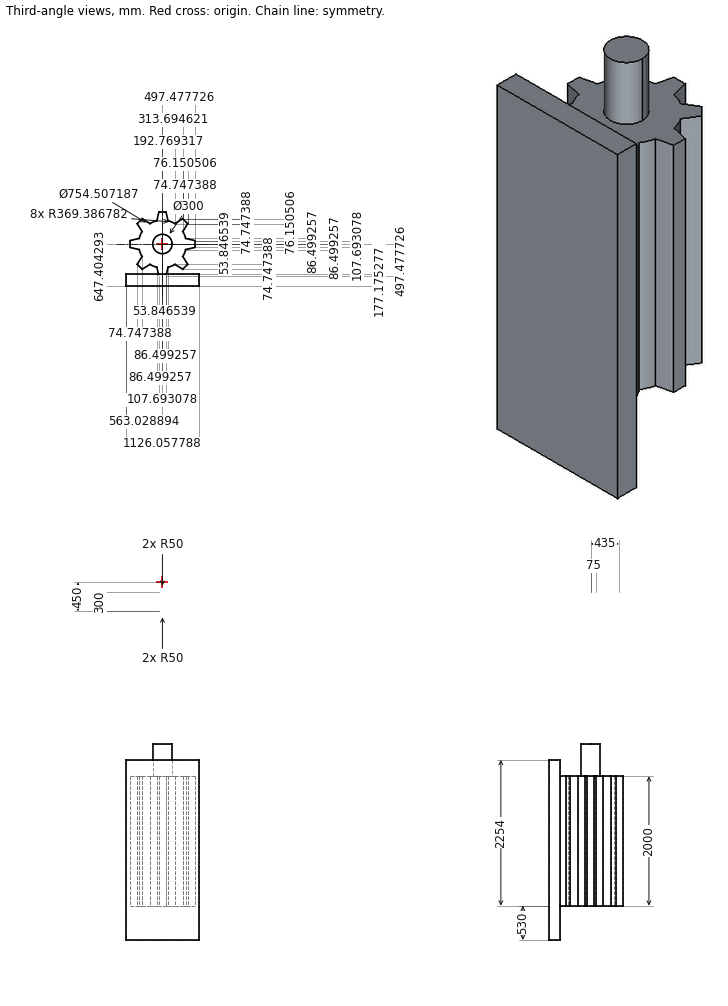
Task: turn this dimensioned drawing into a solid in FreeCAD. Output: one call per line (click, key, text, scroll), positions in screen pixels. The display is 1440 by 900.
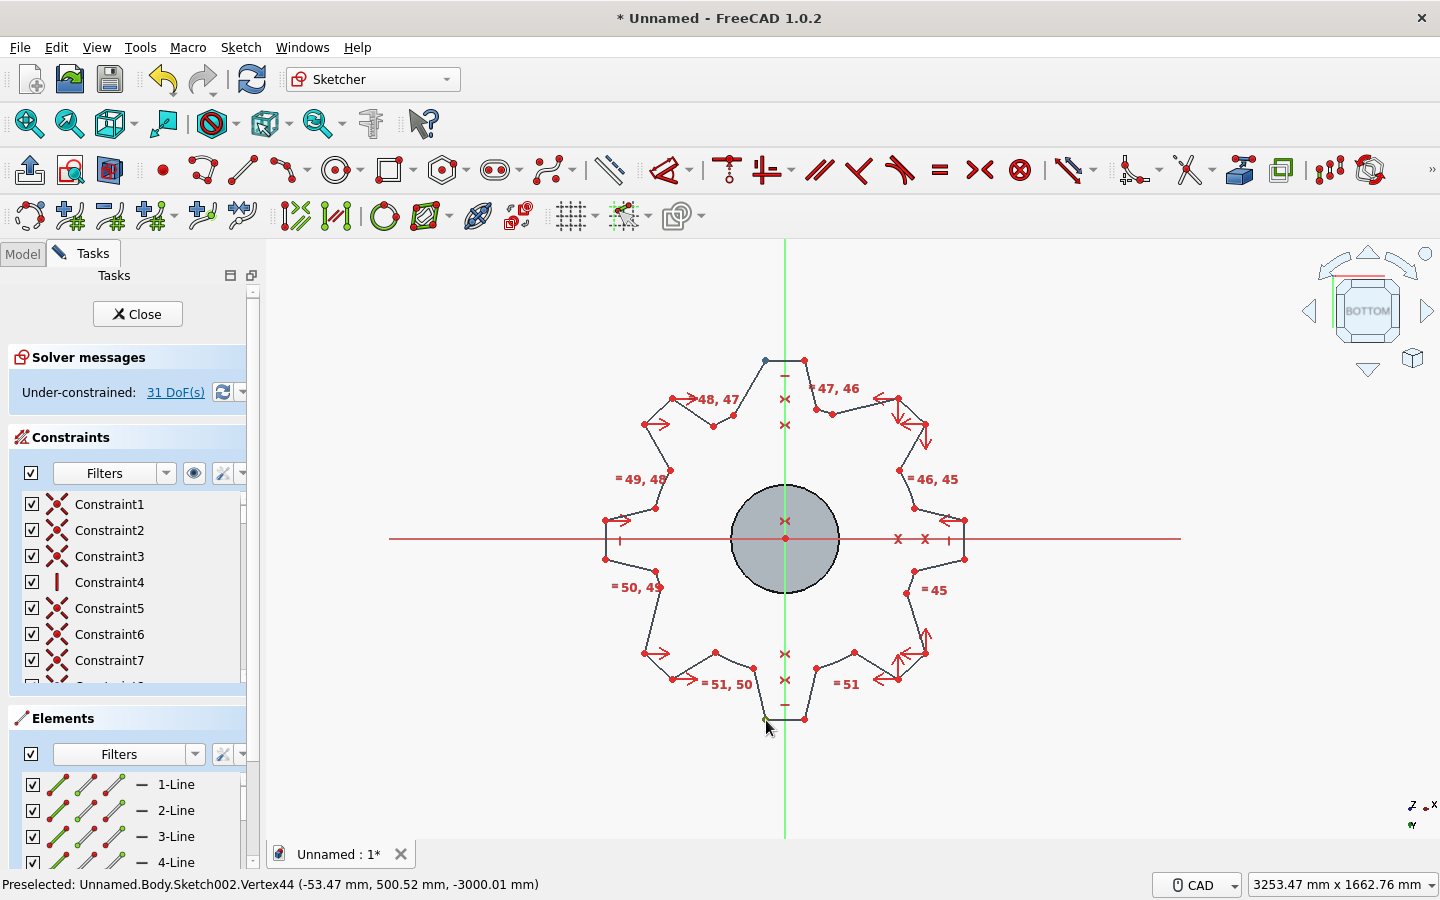
click(434, 539)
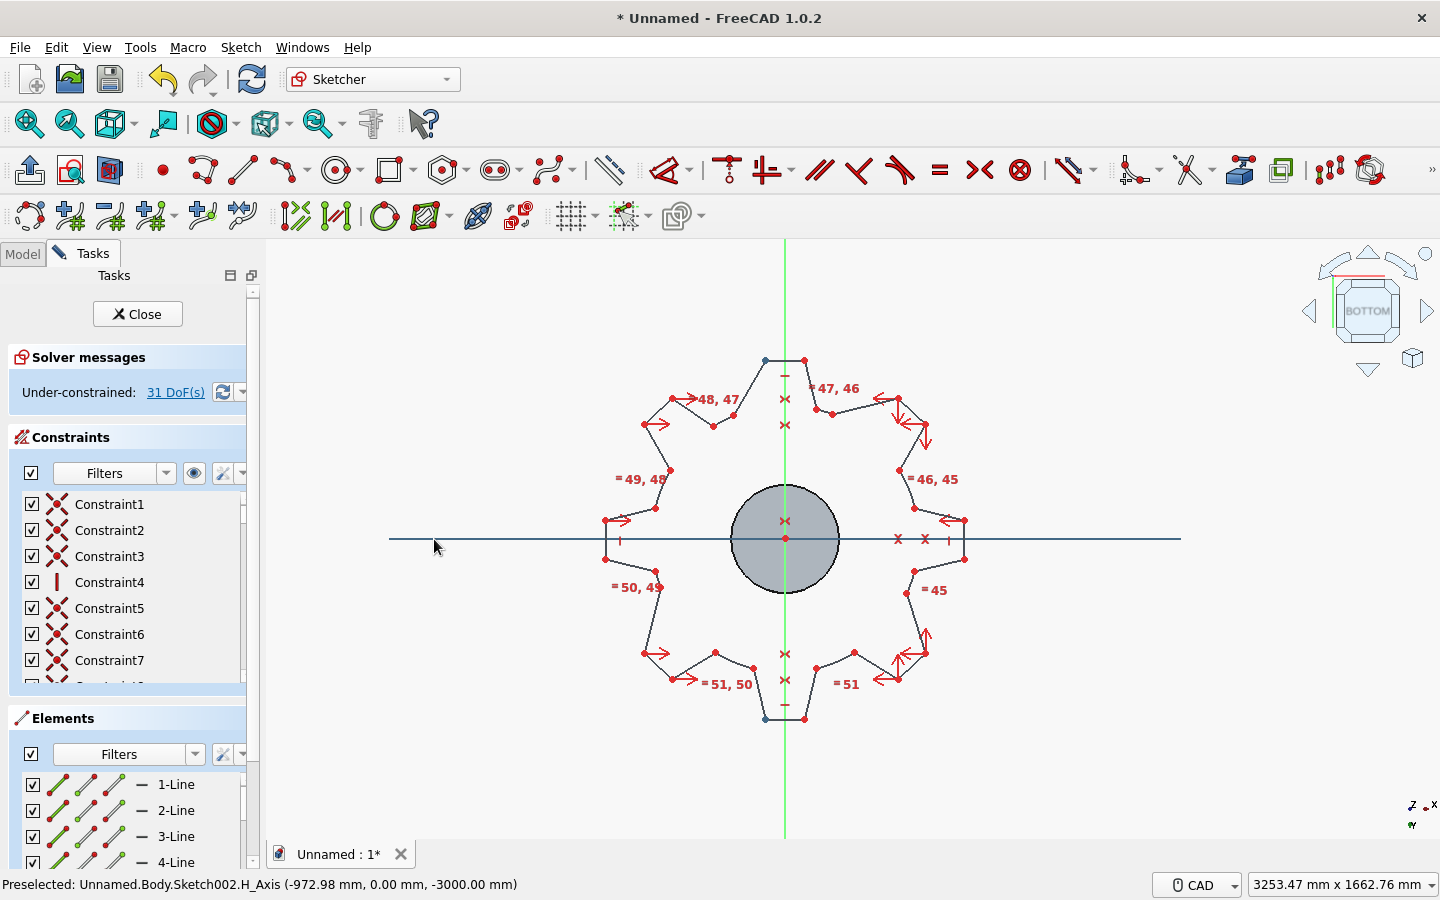
click(980, 170)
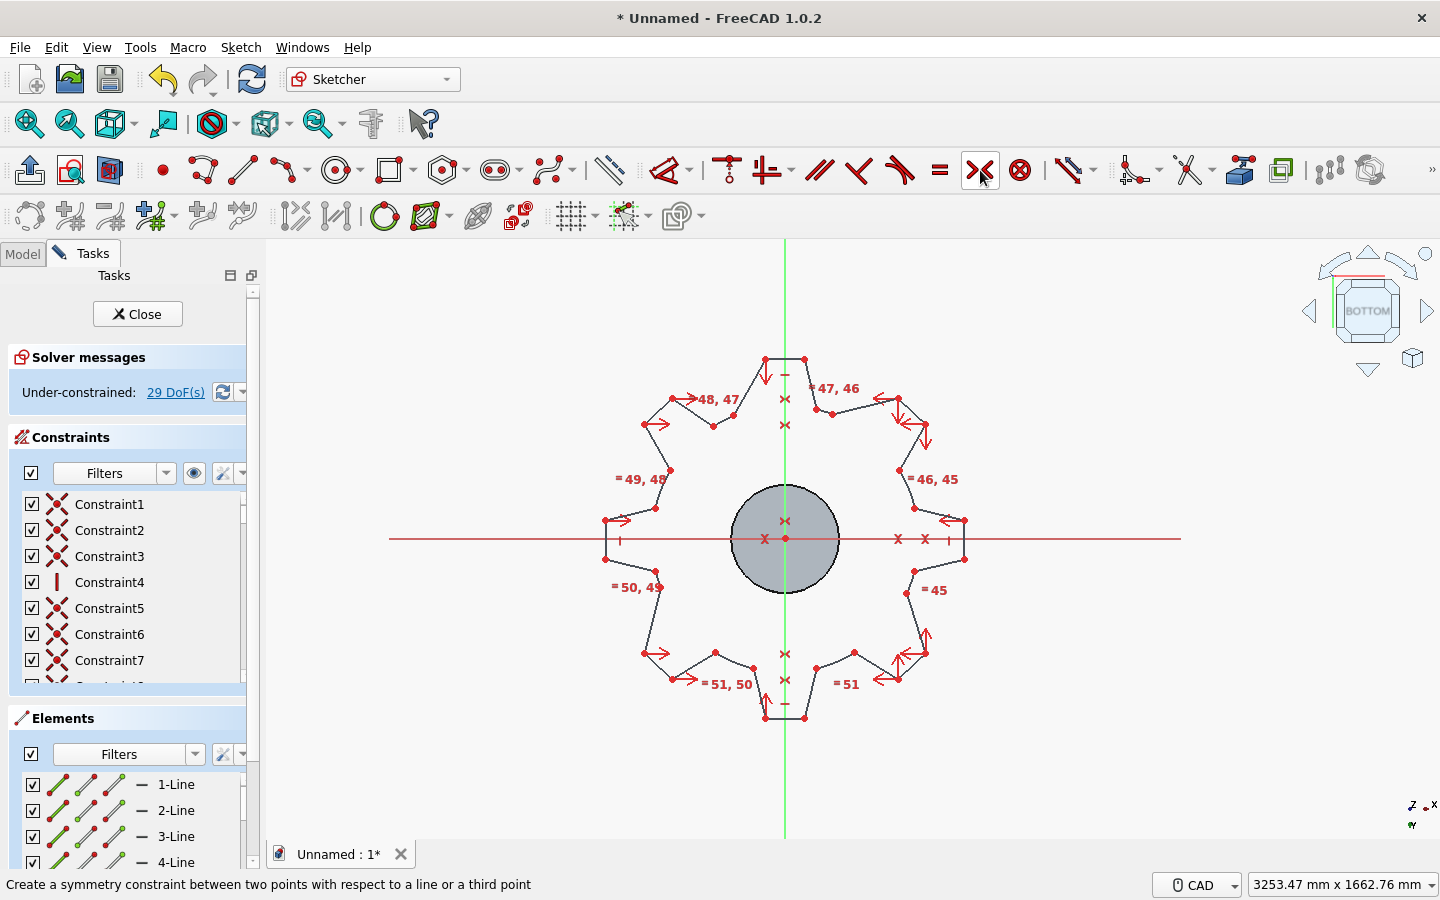
click(664, 170)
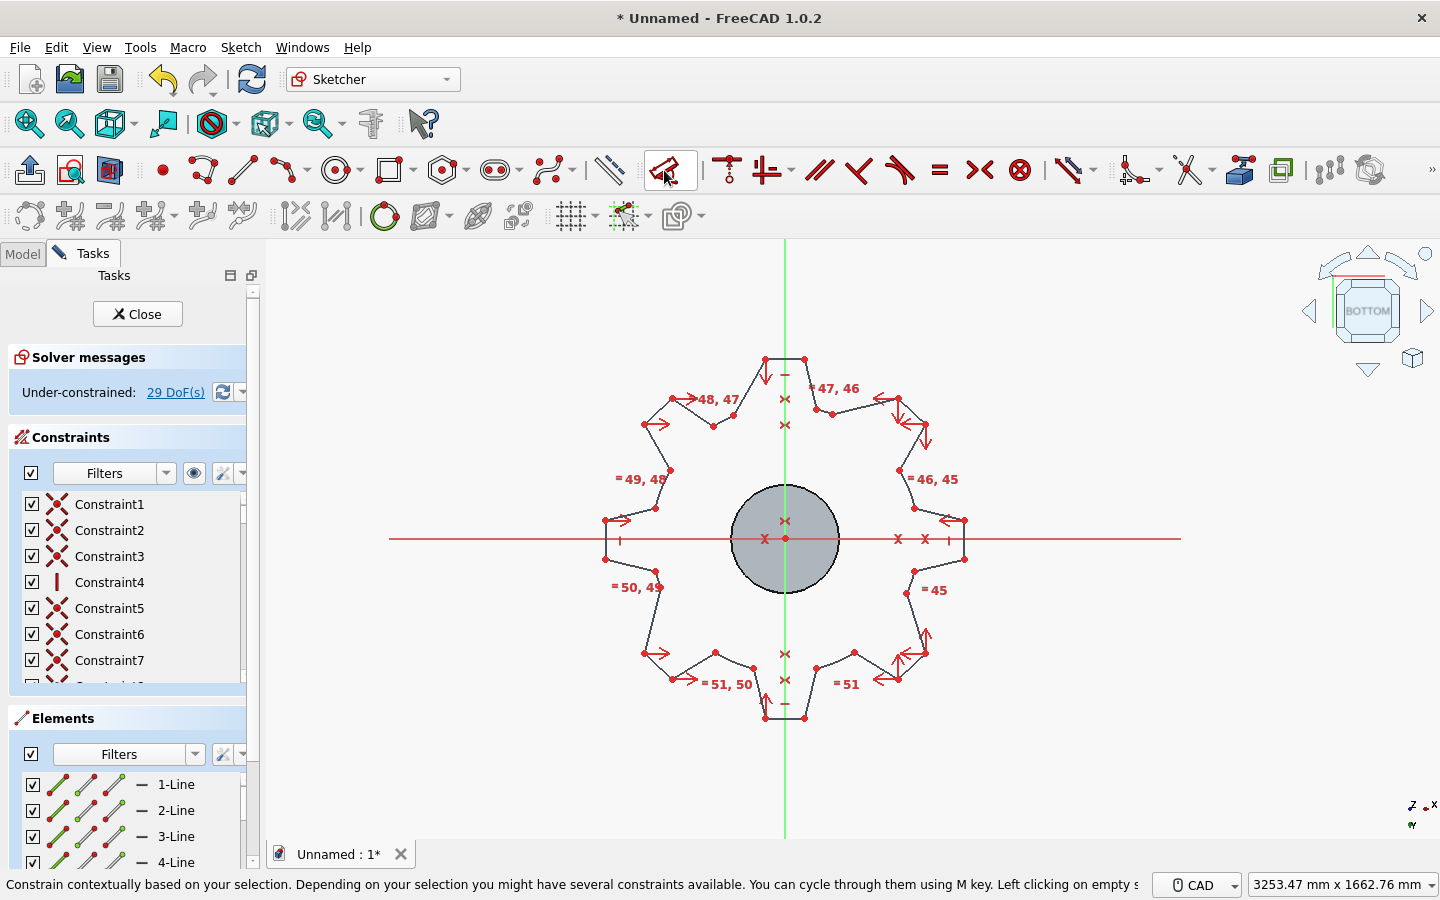
click(911, 583)
click(941, 594)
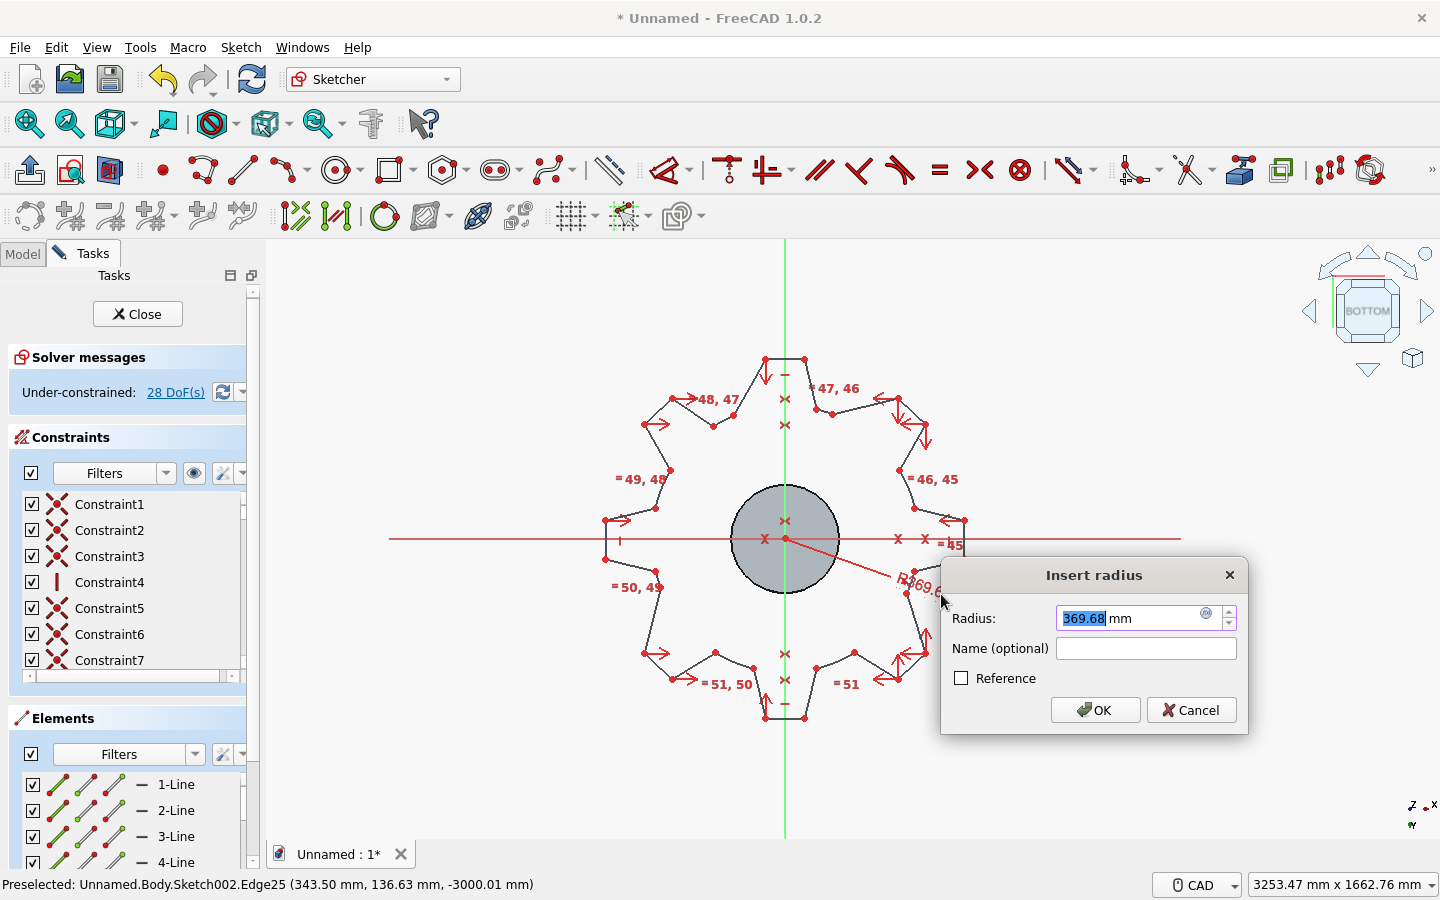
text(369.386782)
key(Return)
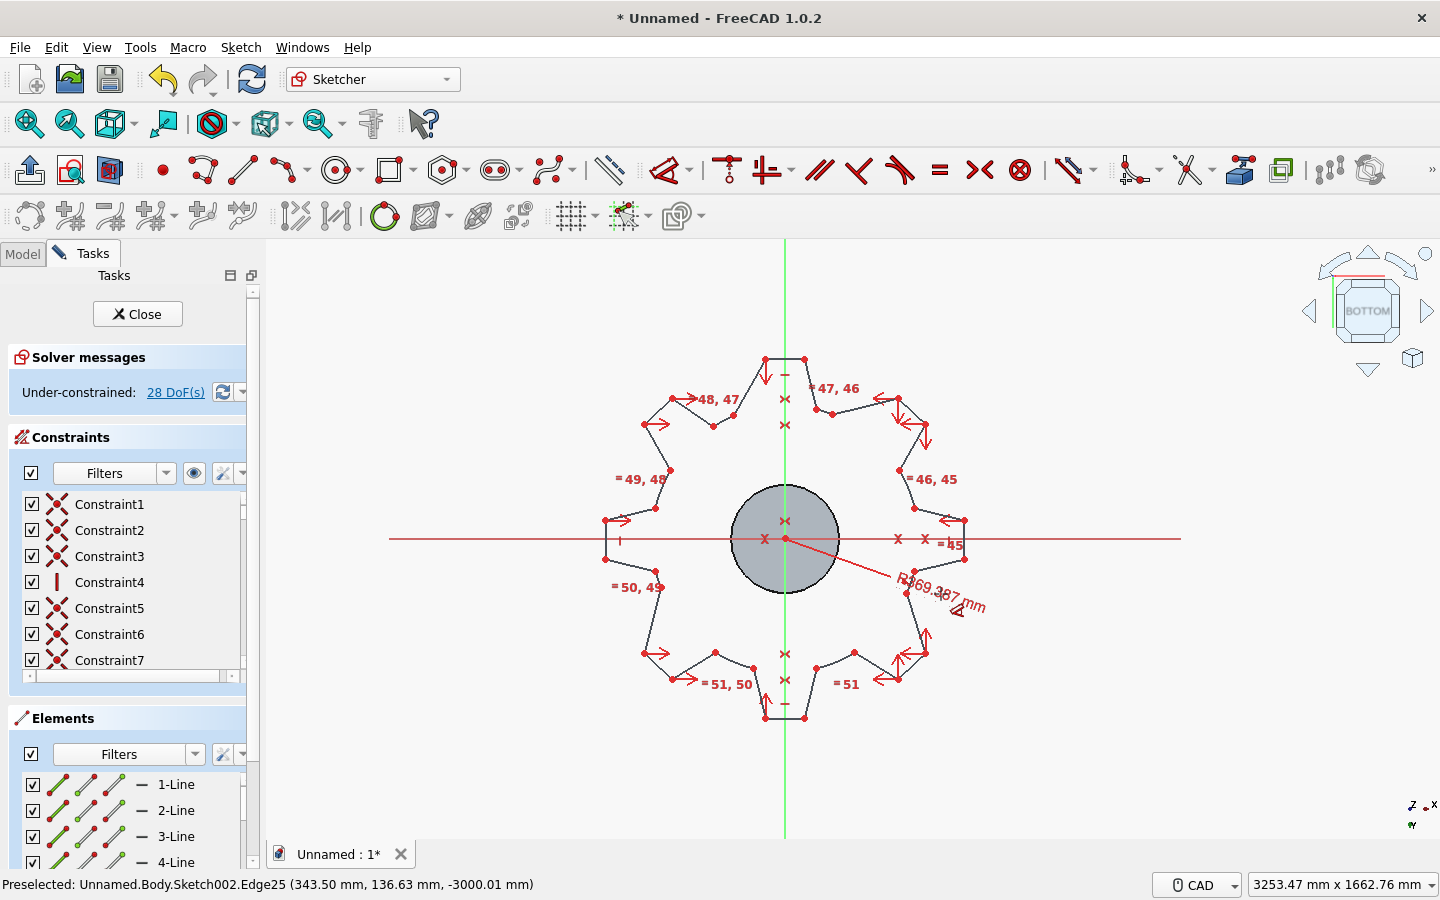
click(964, 536)
click(998, 554)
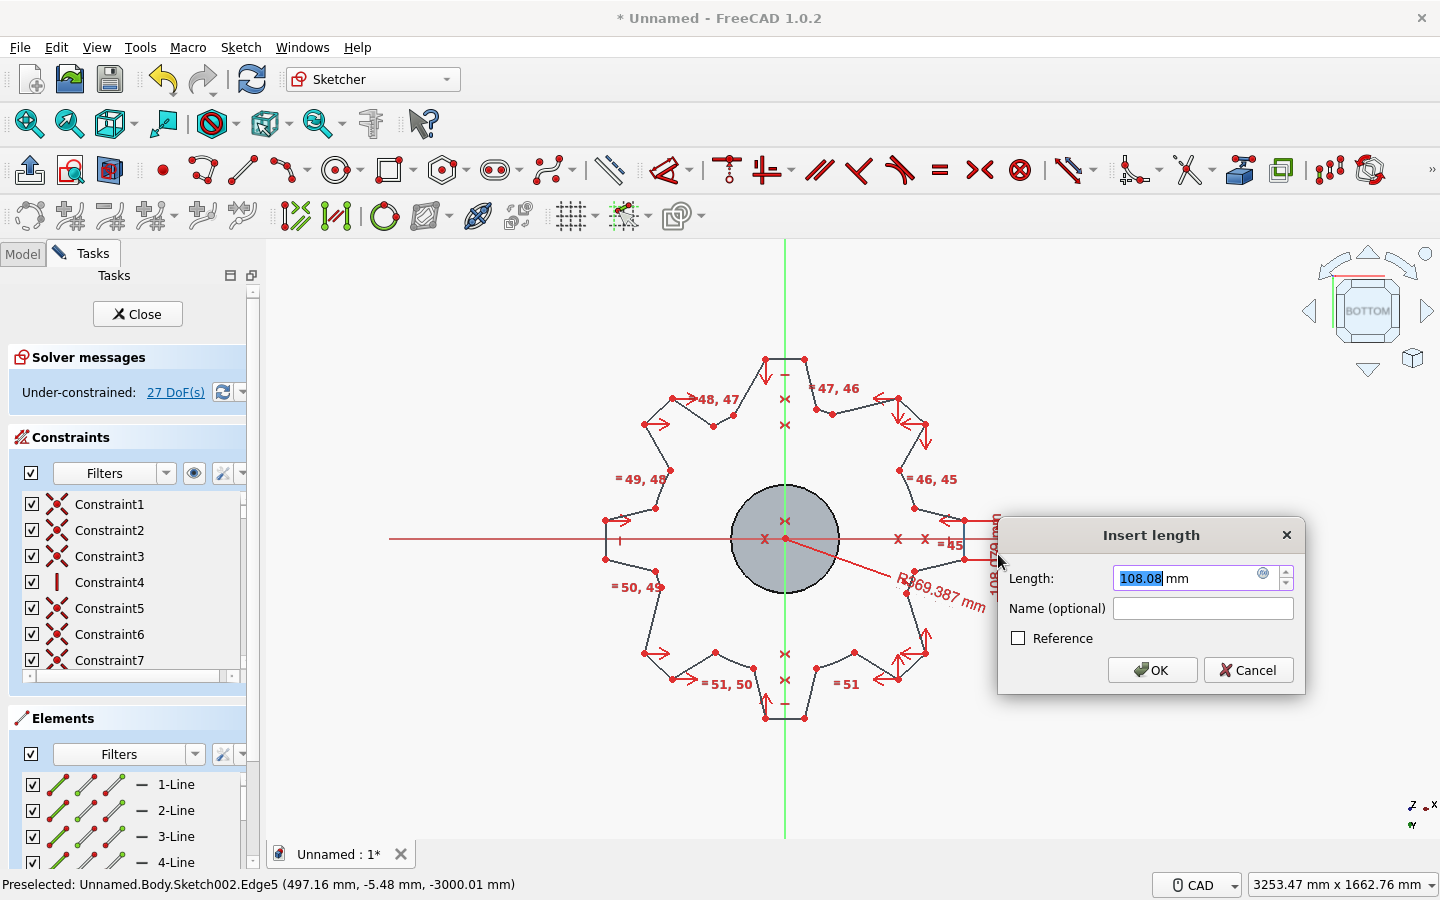
text(107.693078)
key(Return)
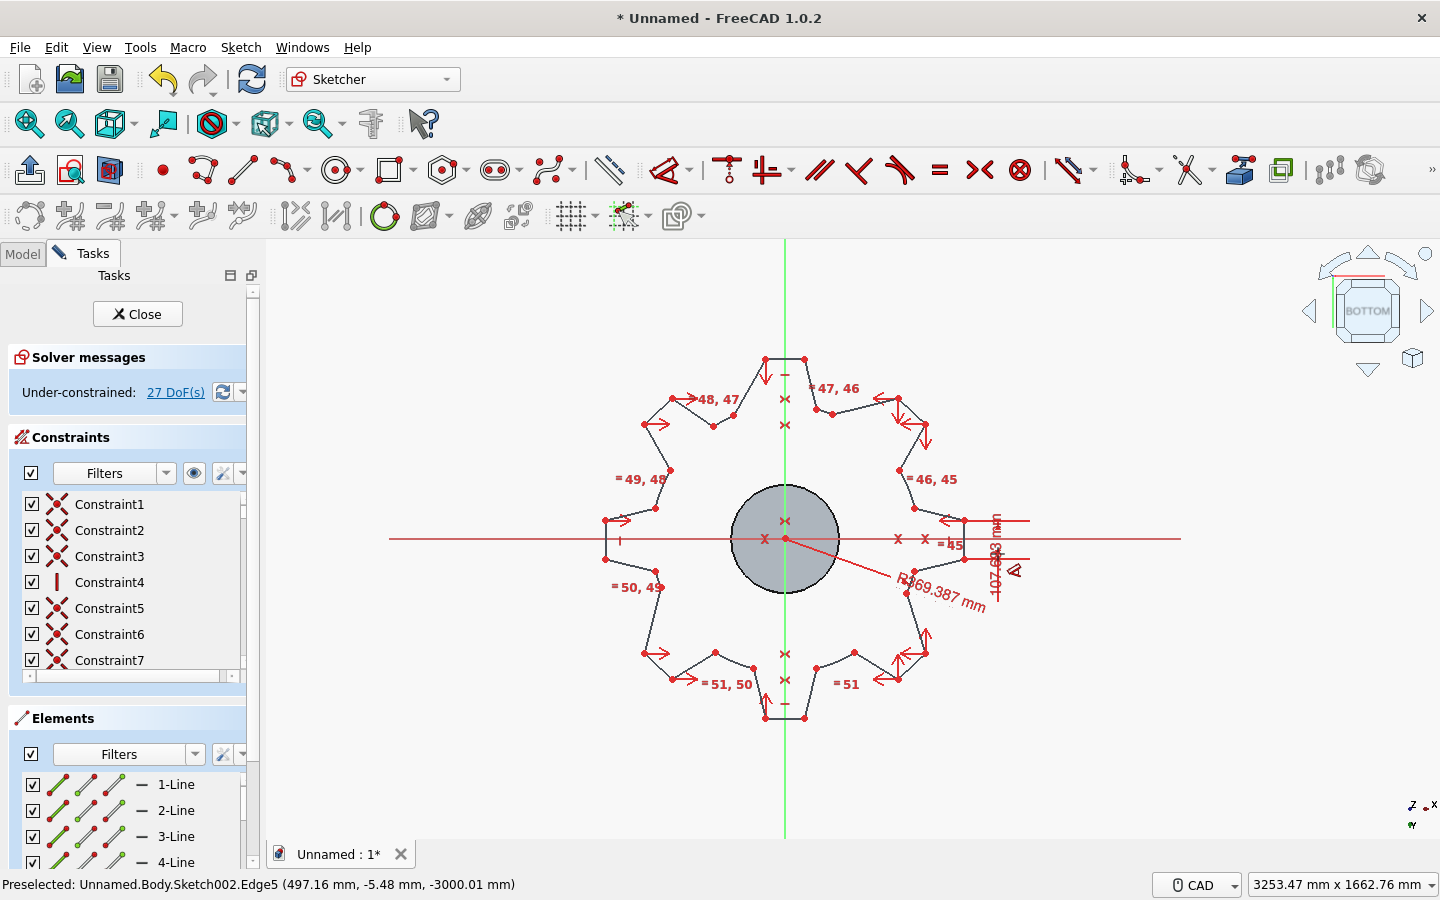
click(781, 359)
click(772, 325)